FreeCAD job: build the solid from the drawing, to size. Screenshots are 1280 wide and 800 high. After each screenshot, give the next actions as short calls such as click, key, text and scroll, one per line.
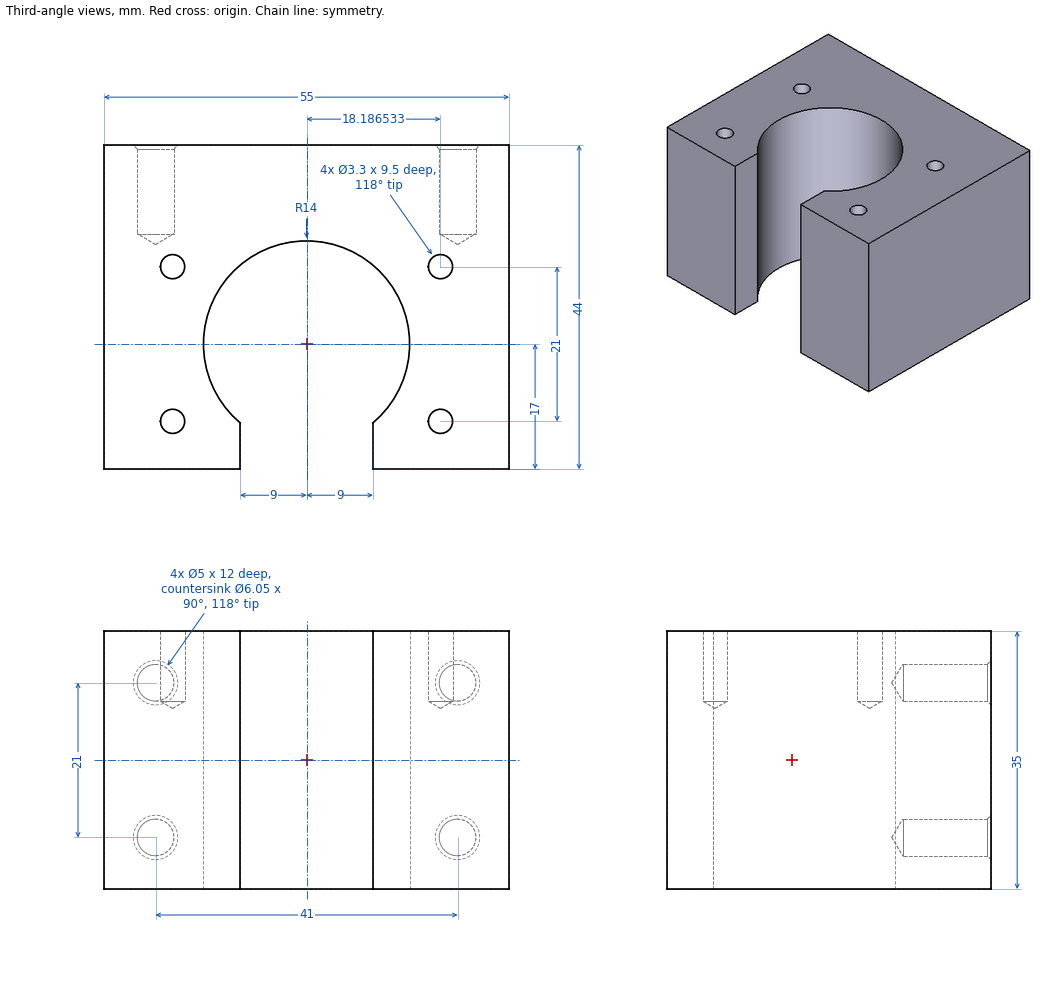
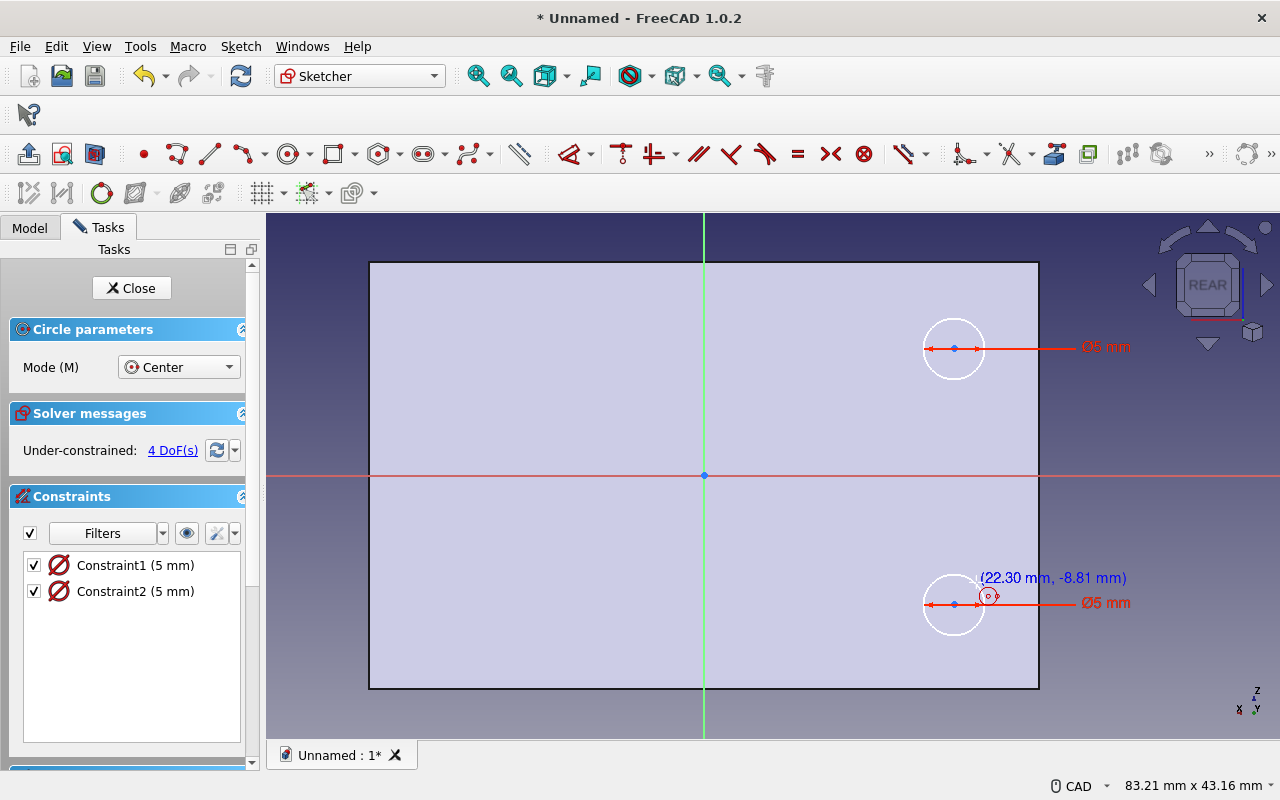
click(454, 604)
move(476, 582)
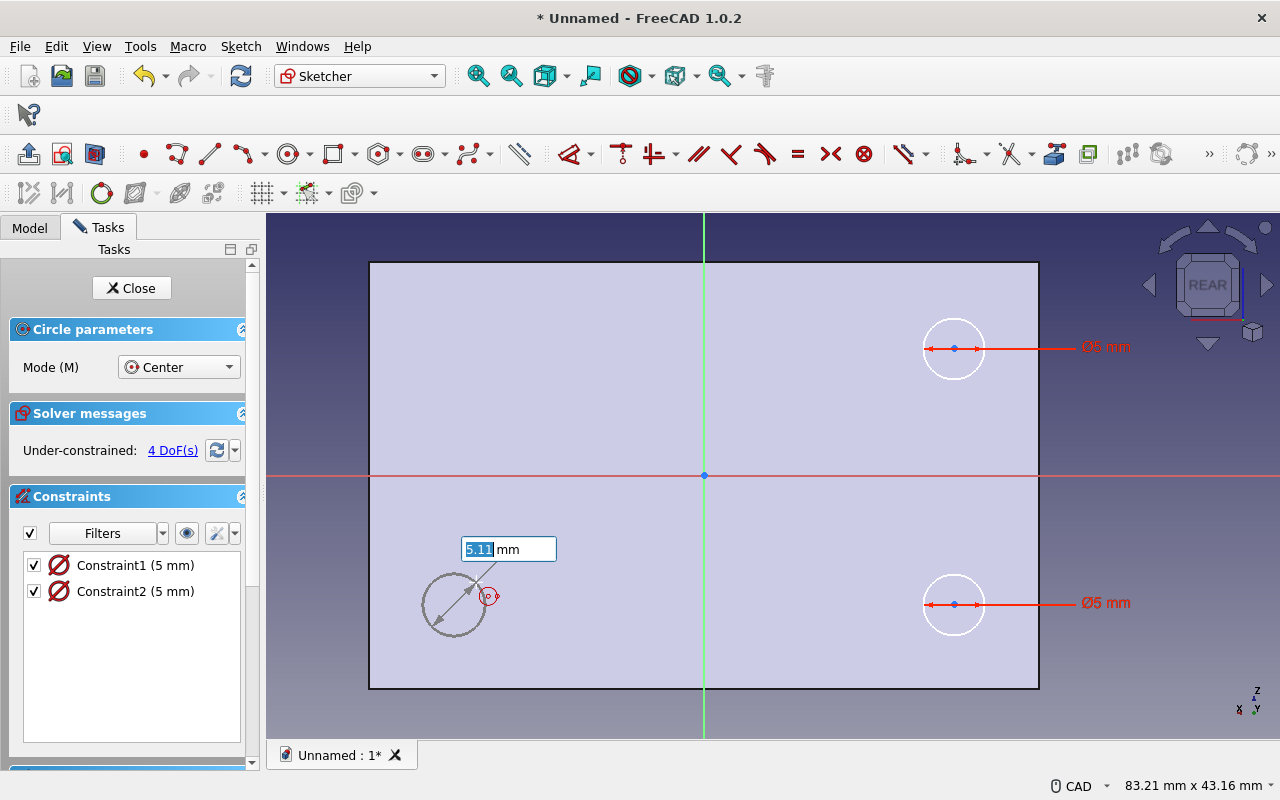
text(5)
key(Return)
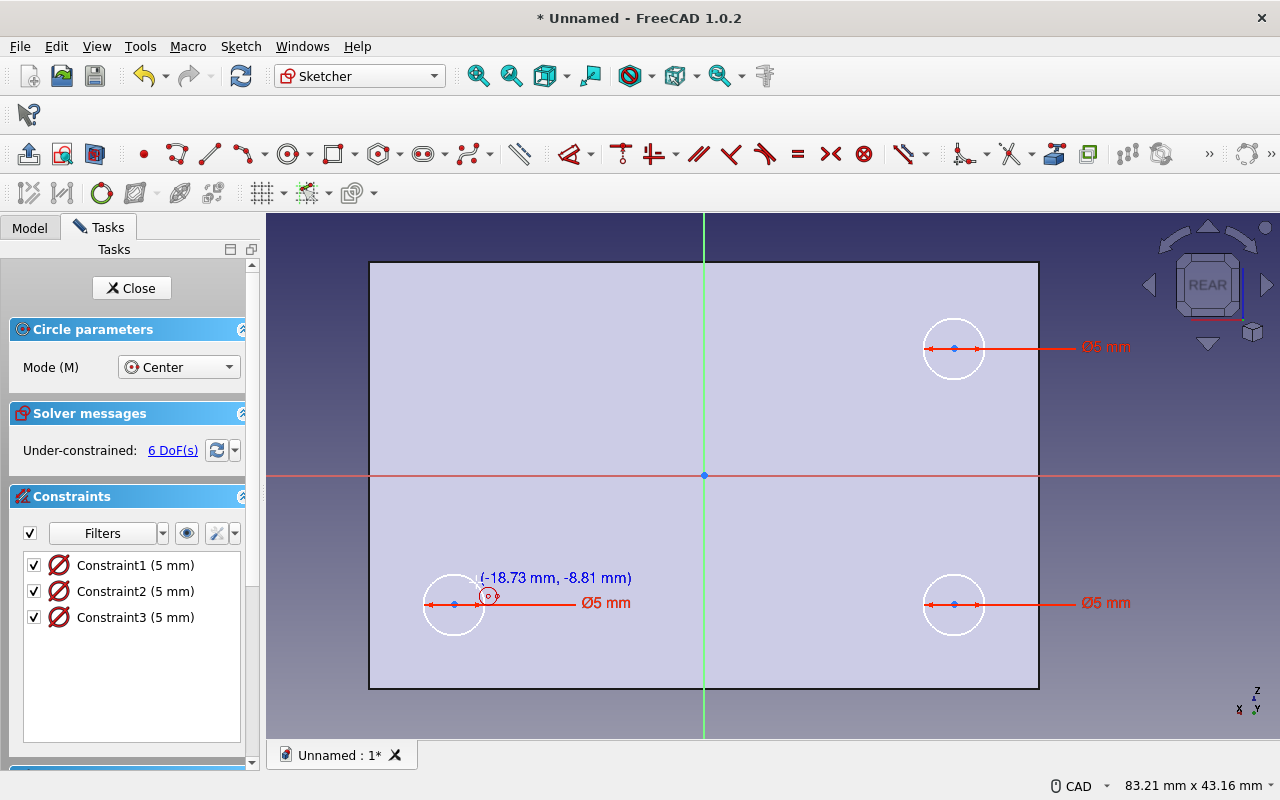
click(454, 348)
move(476, 326)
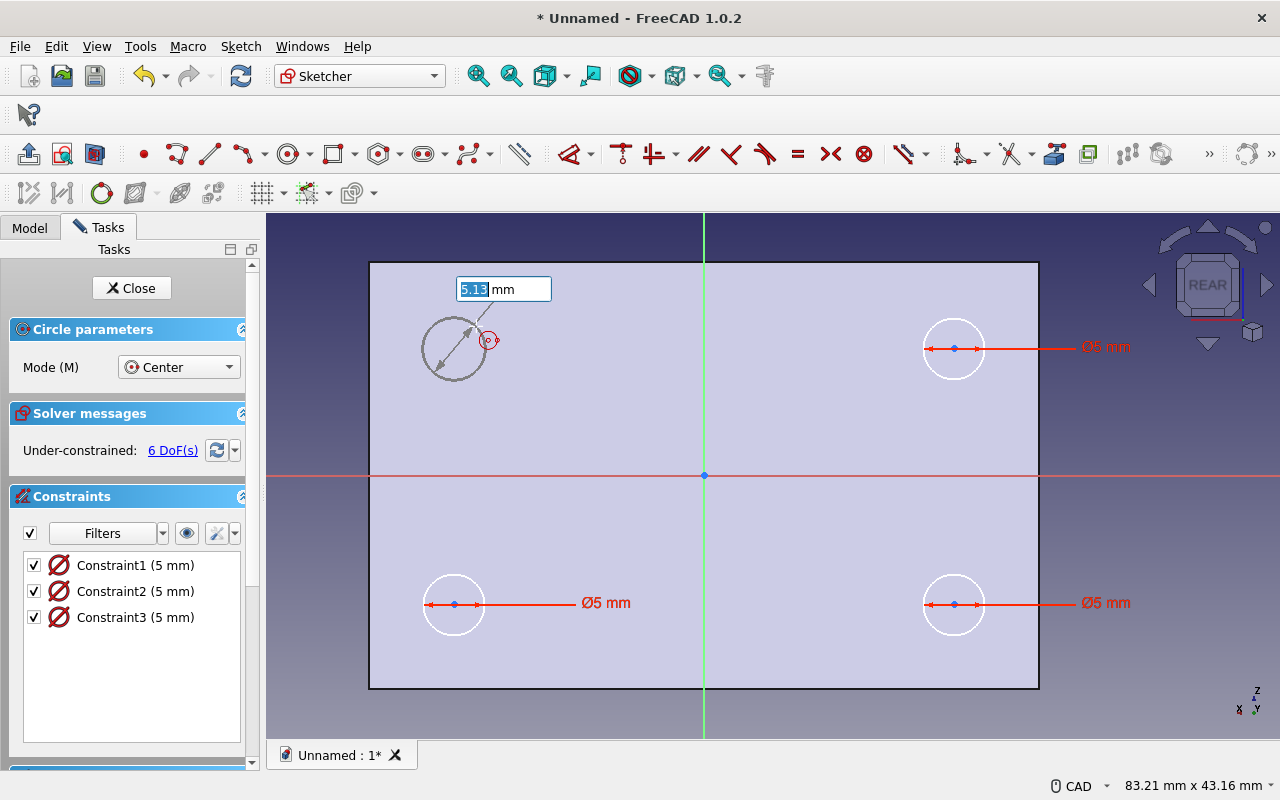
text(5)
key(Return)
key(Escape)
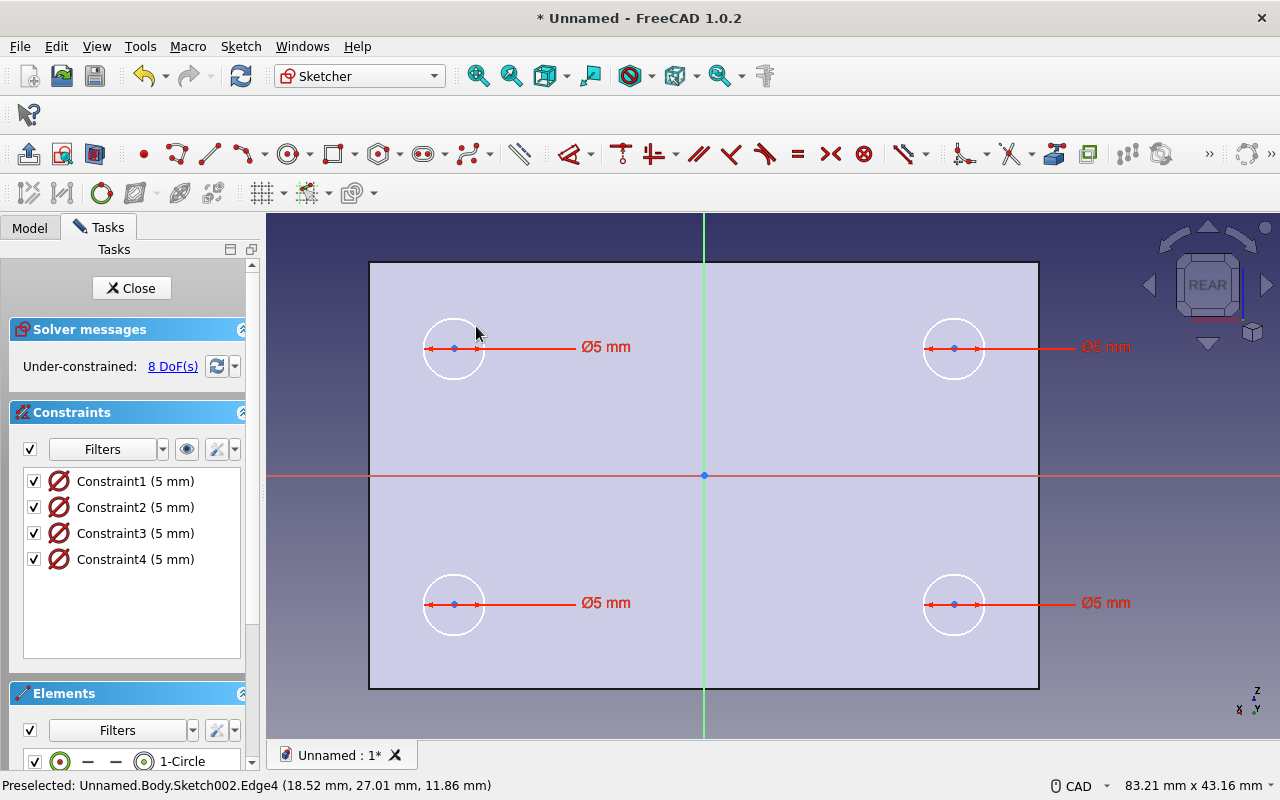
click(954, 349)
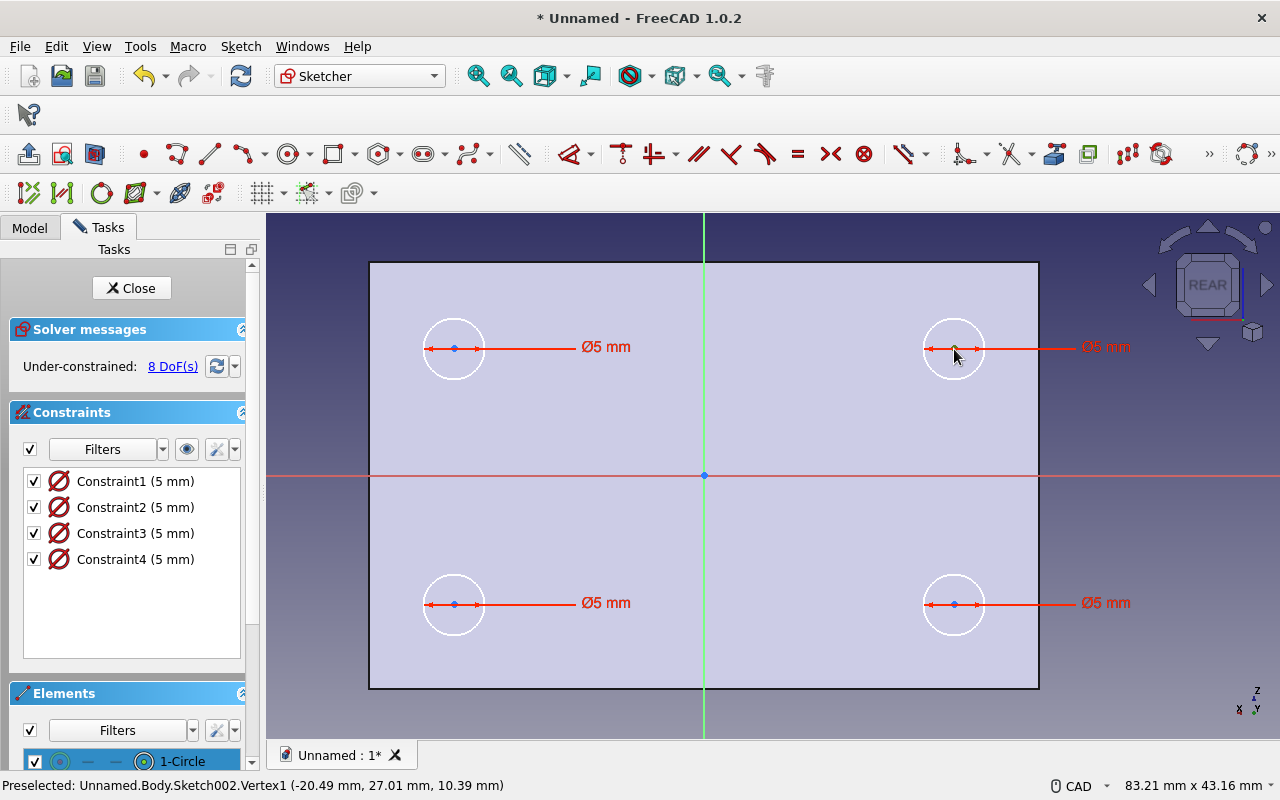
click(954, 605)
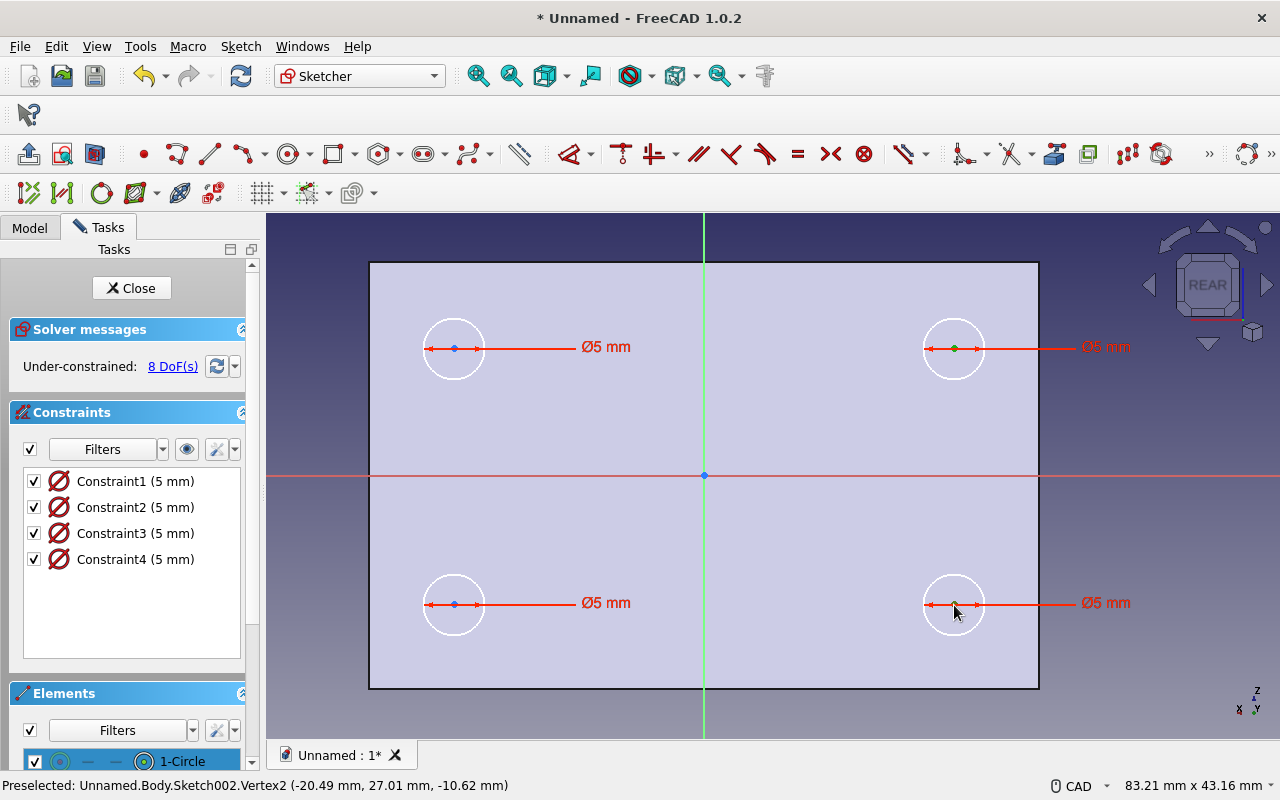
click(353, 476)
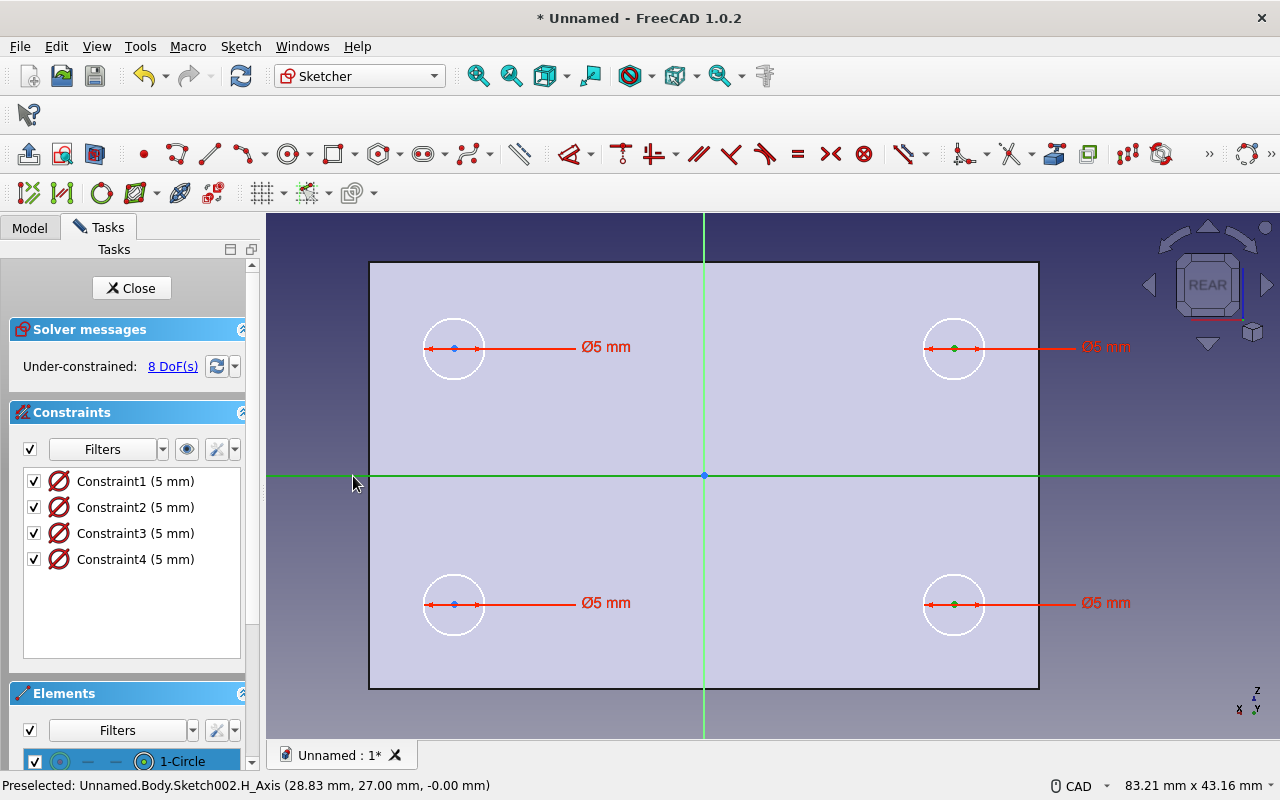
click(831, 154)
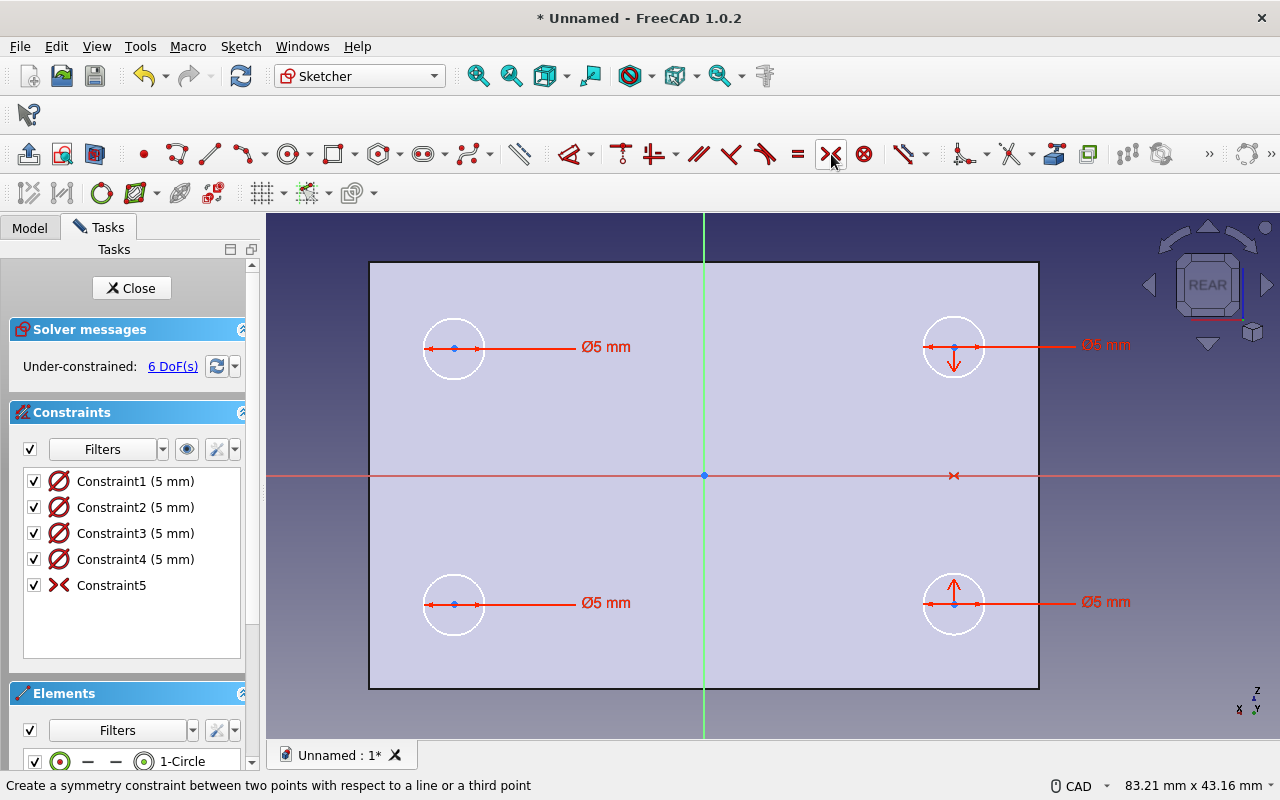
click(954, 604)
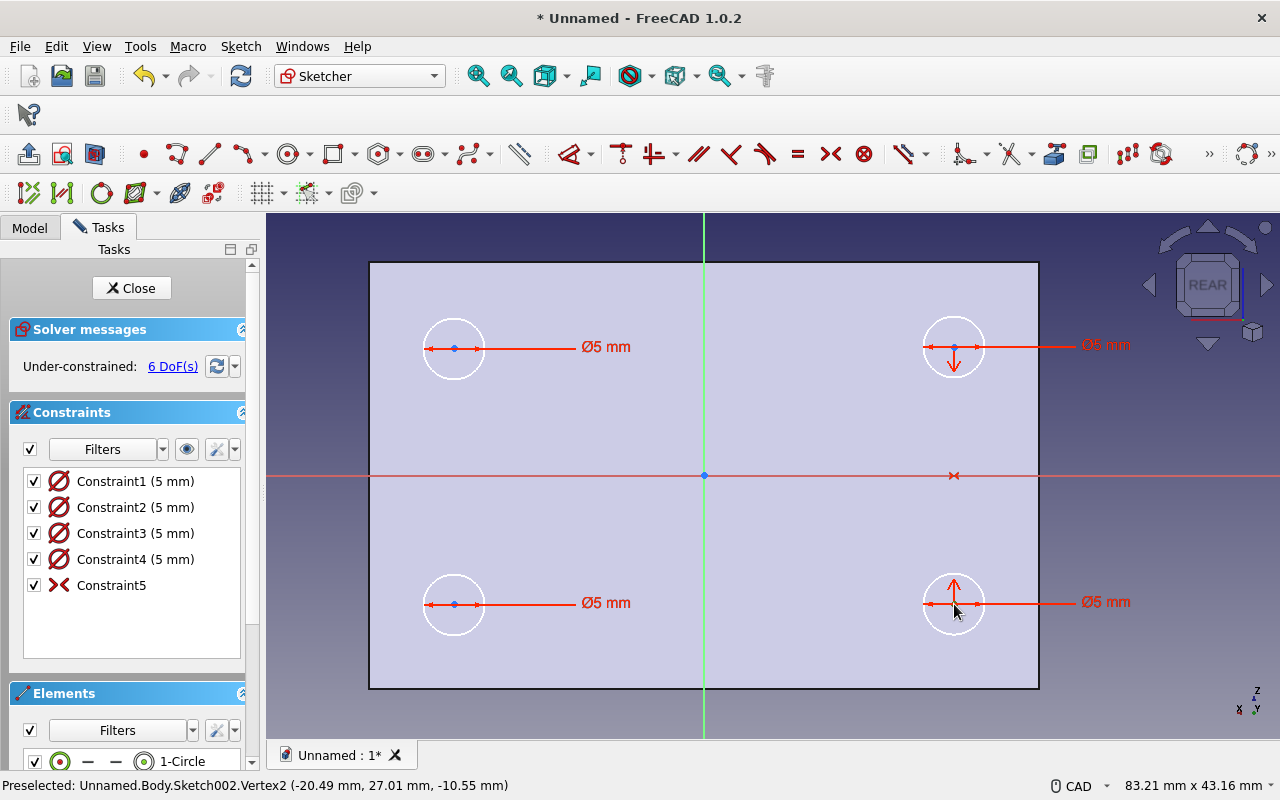
click(454, 605)